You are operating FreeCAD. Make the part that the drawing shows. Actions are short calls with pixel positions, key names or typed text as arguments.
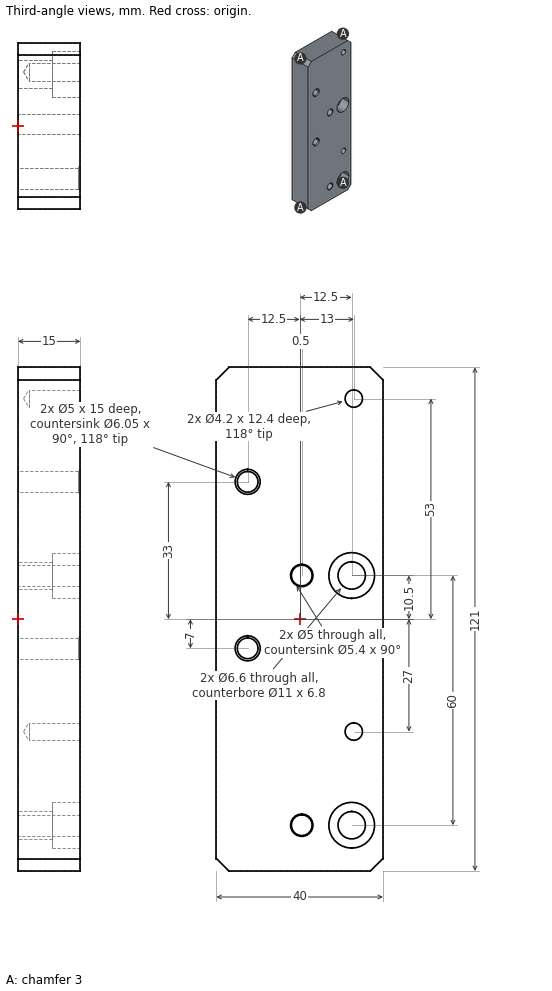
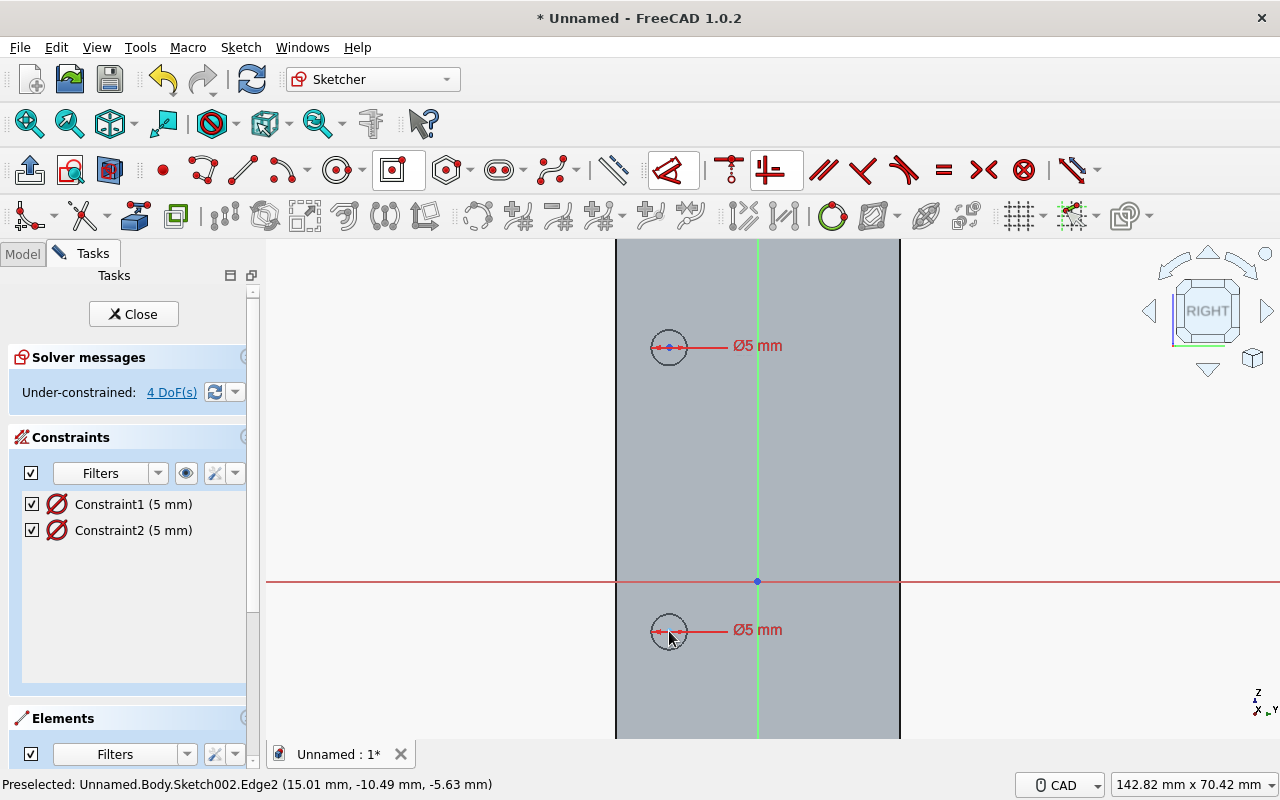
click(669, 348)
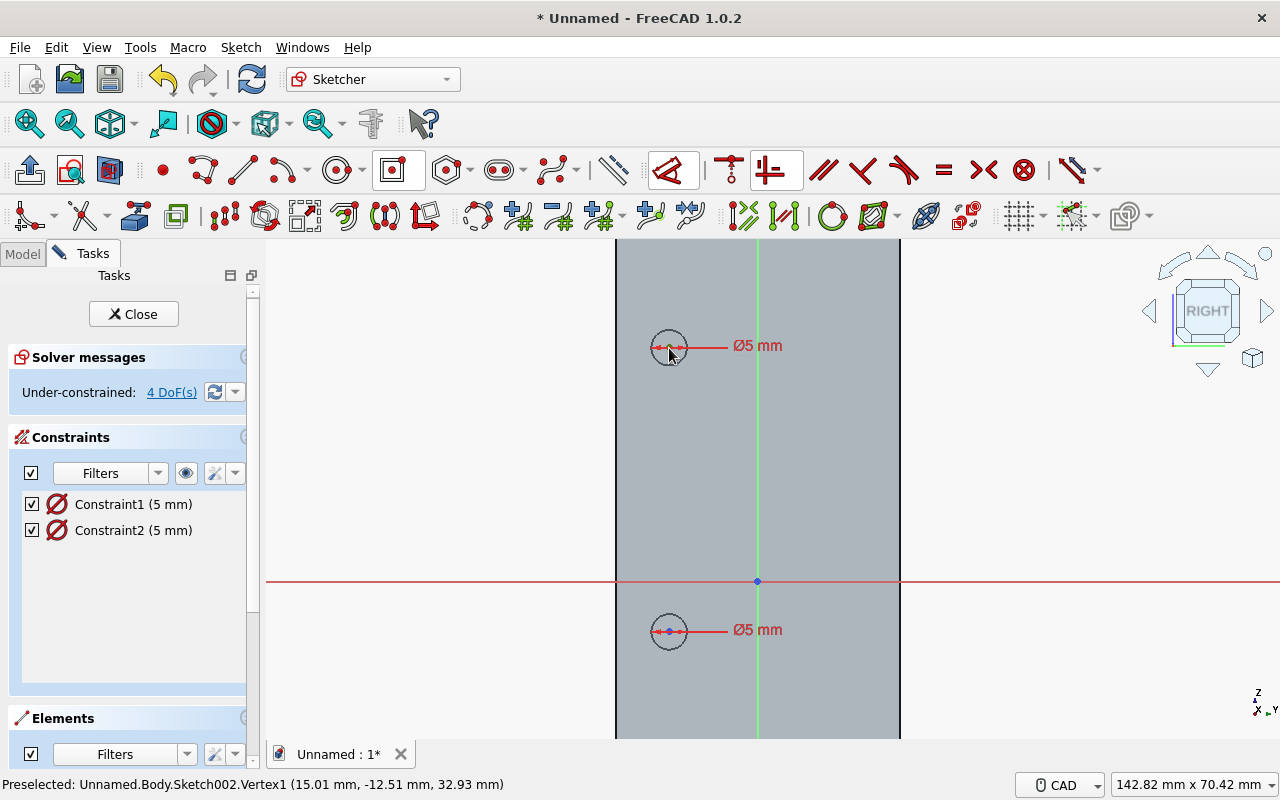
click(669, 632)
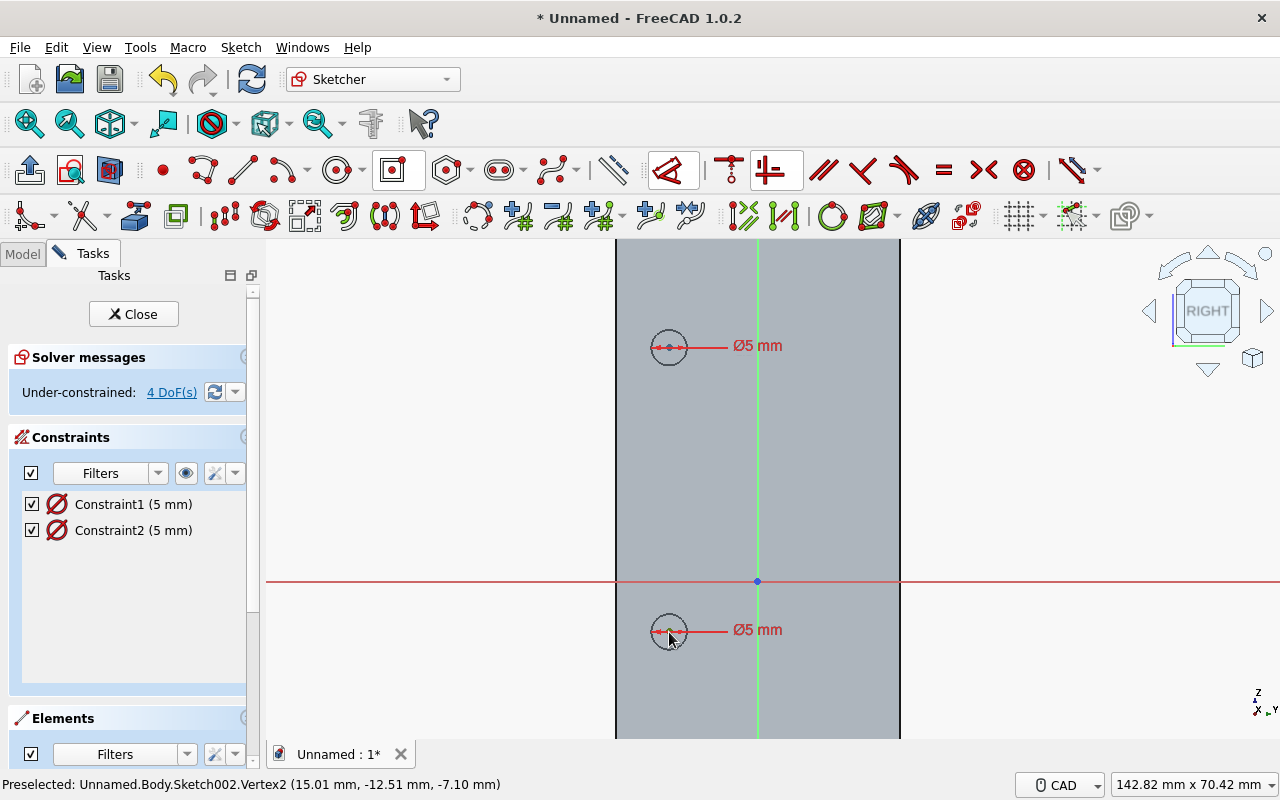
click(798, 170)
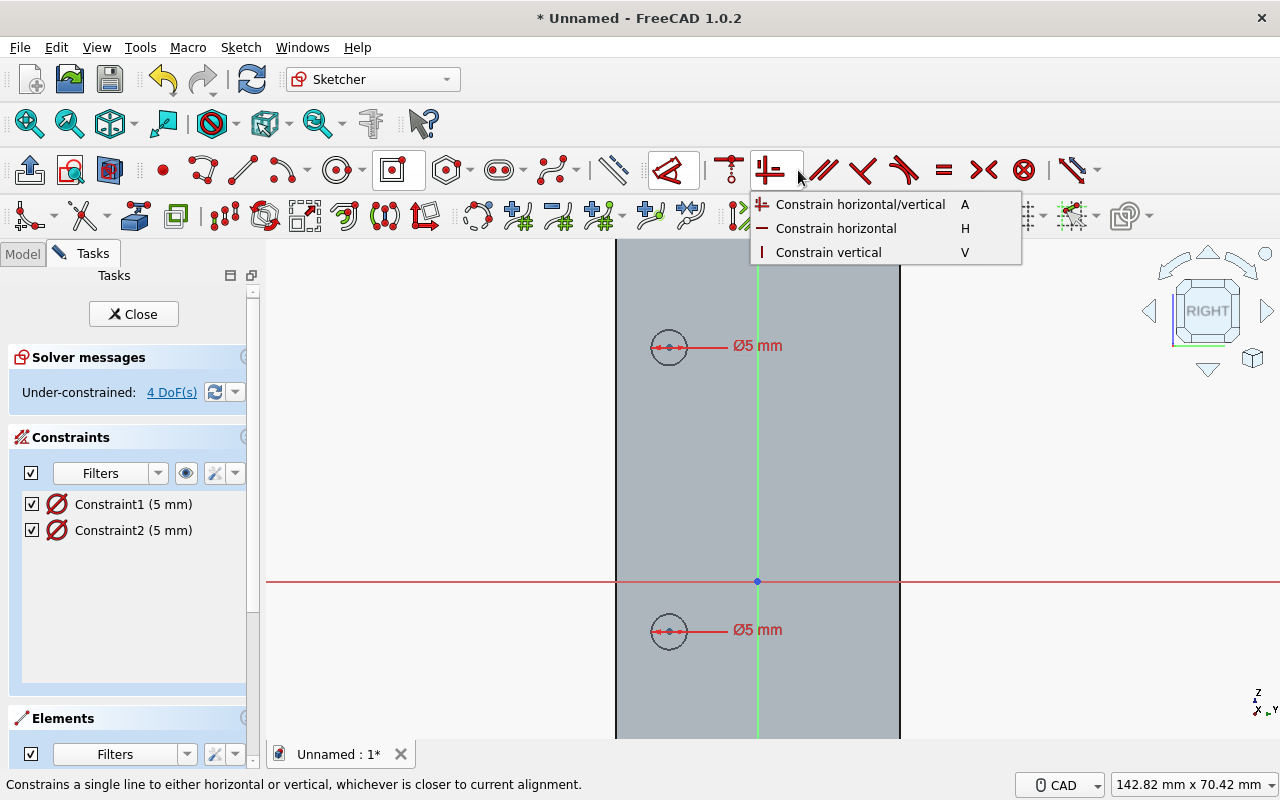
click(886, 252)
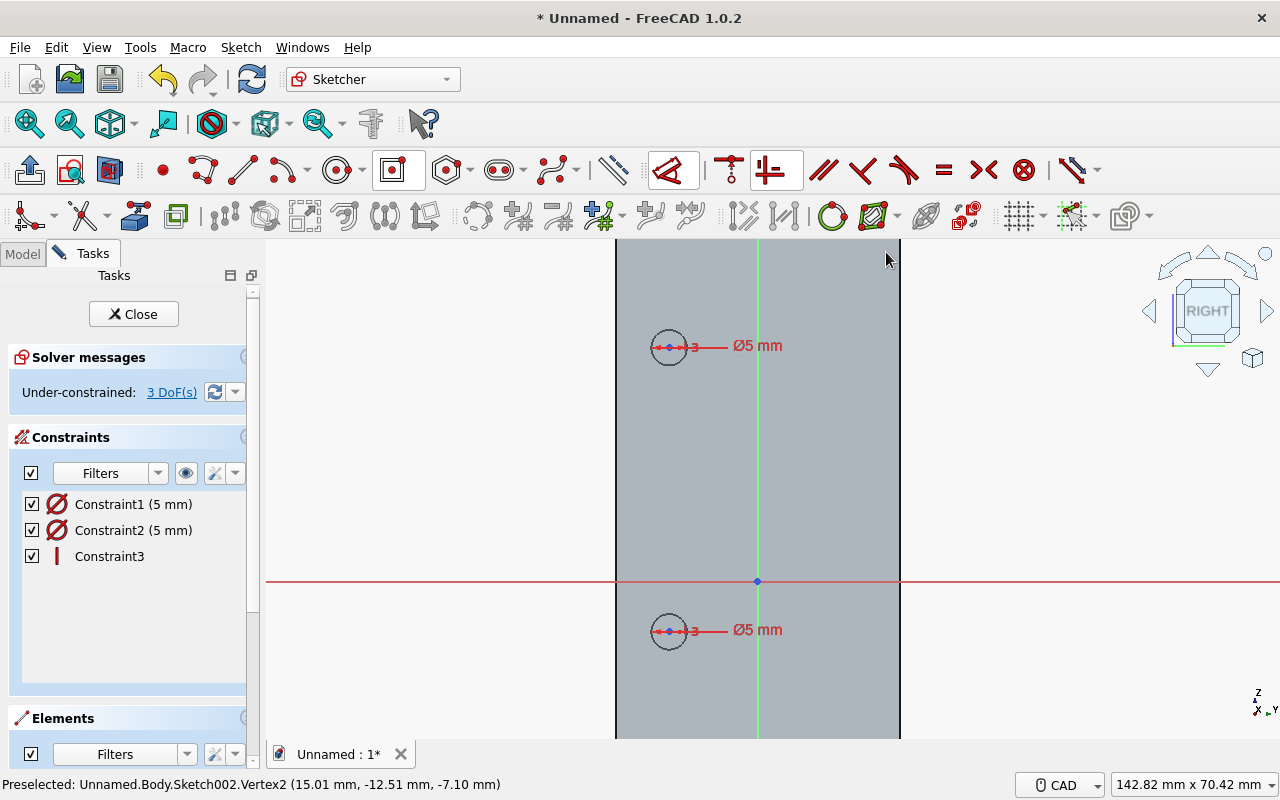
click(669, 632)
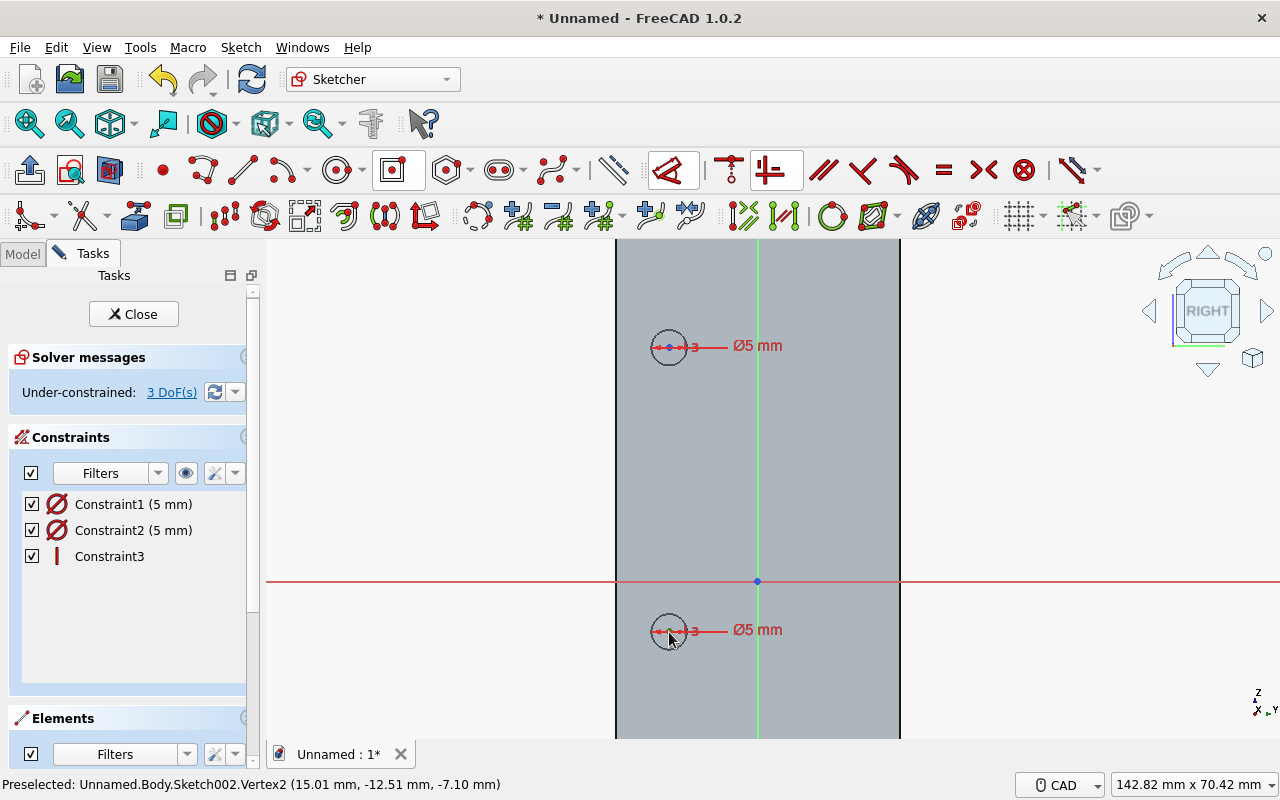
key(i)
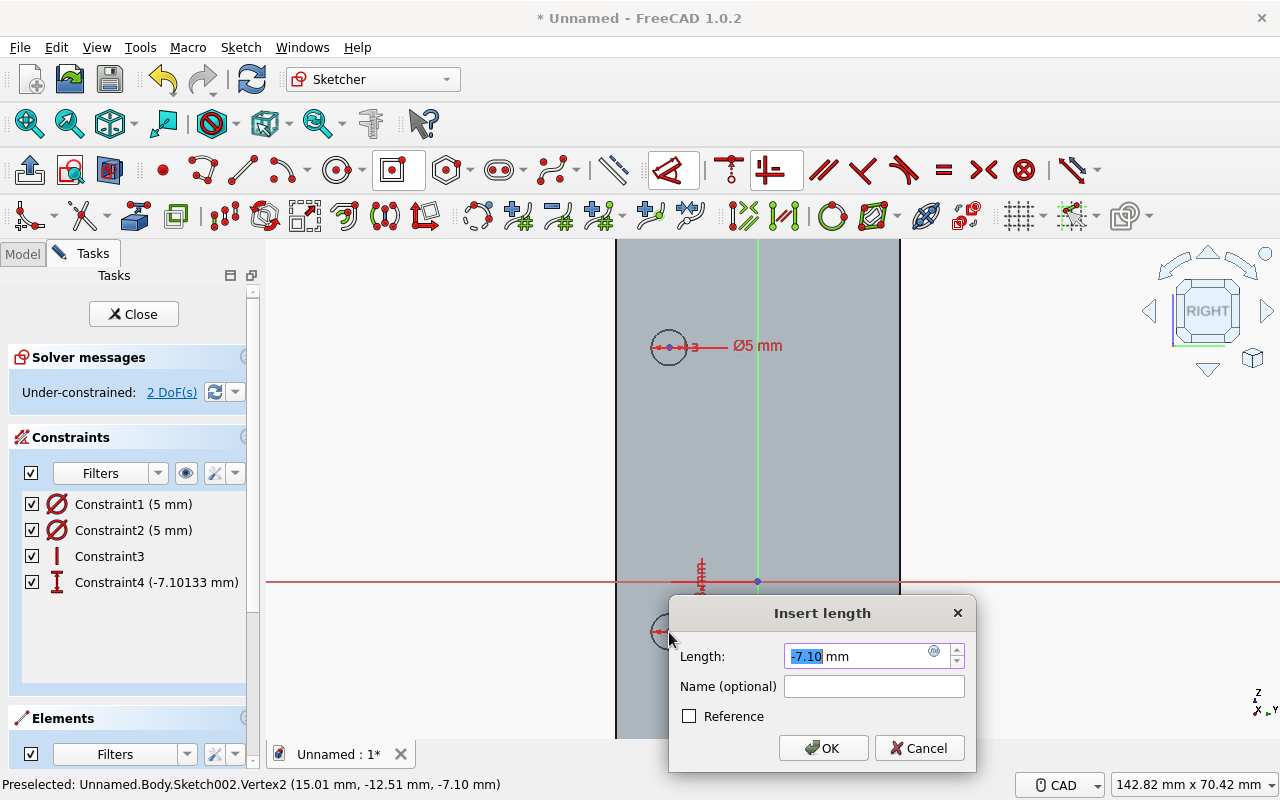
text(-7)
key(Return)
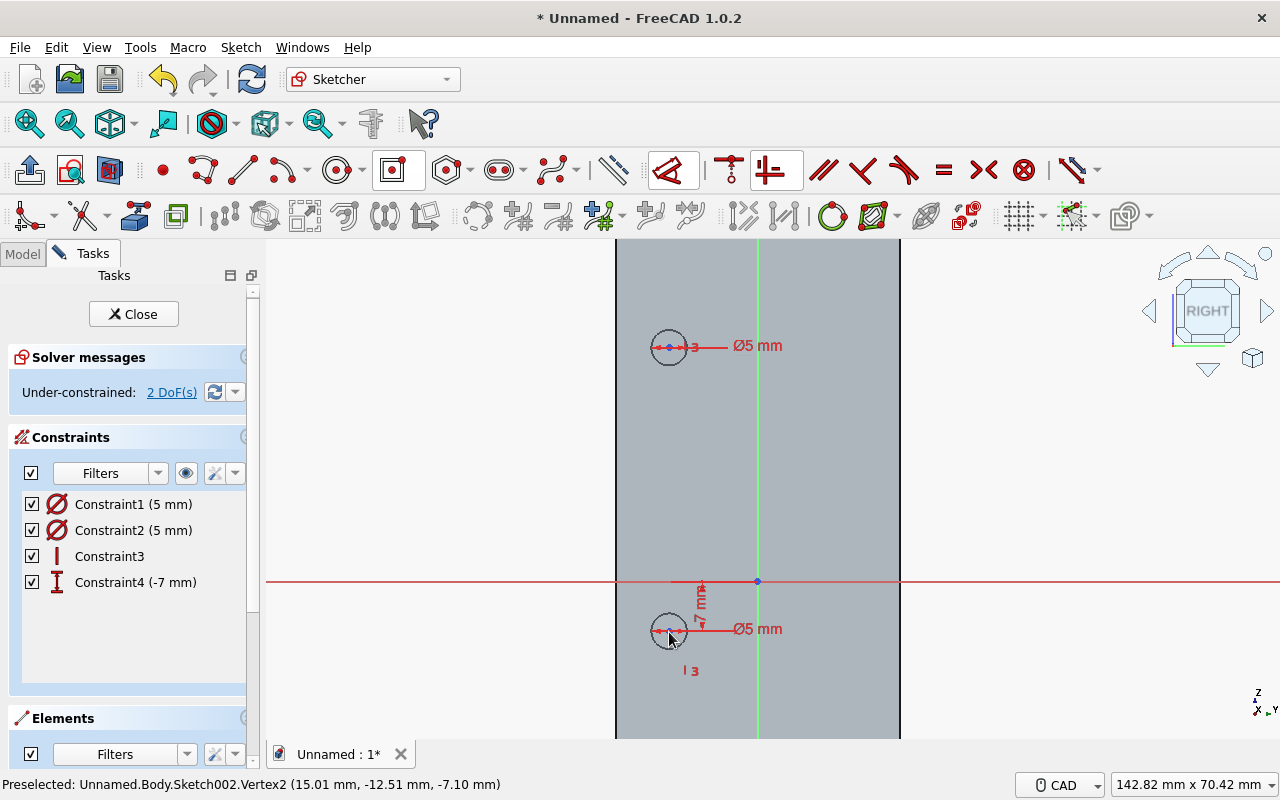
click(669, 348)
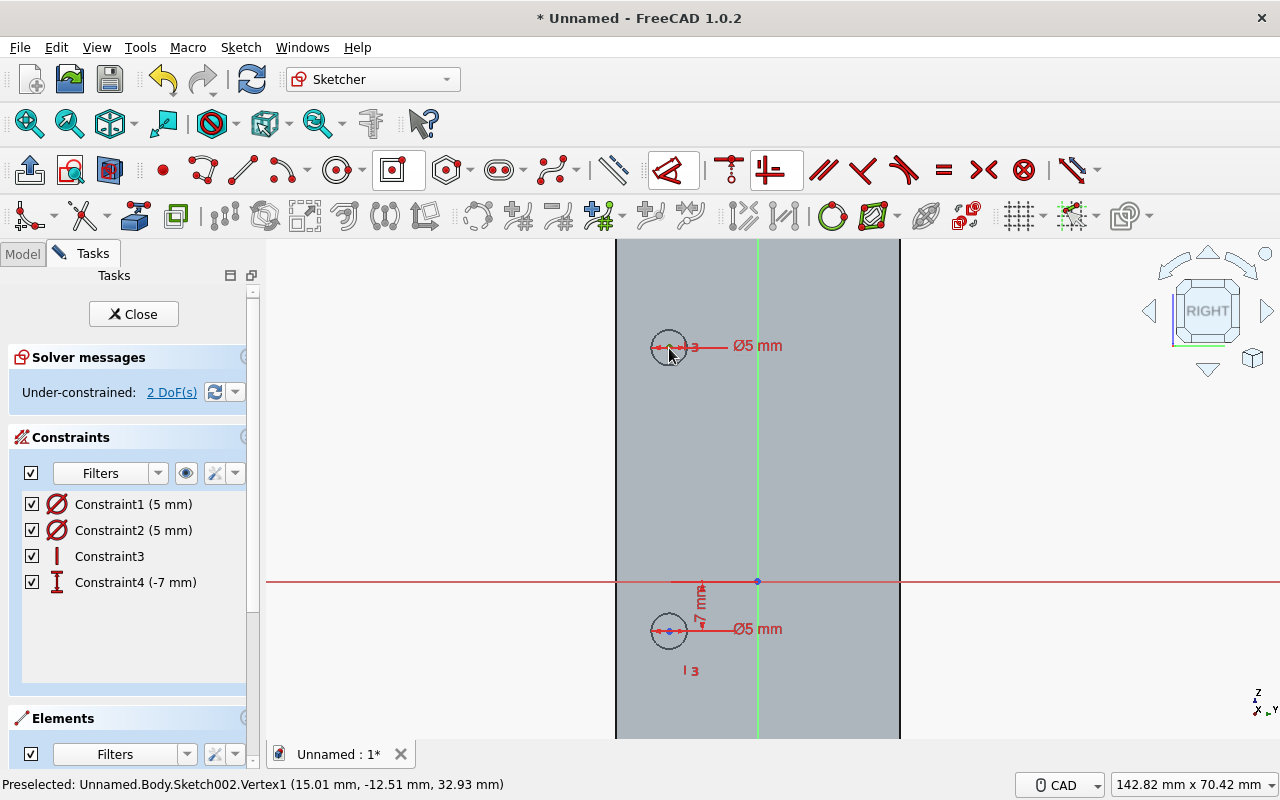
click(694, 170)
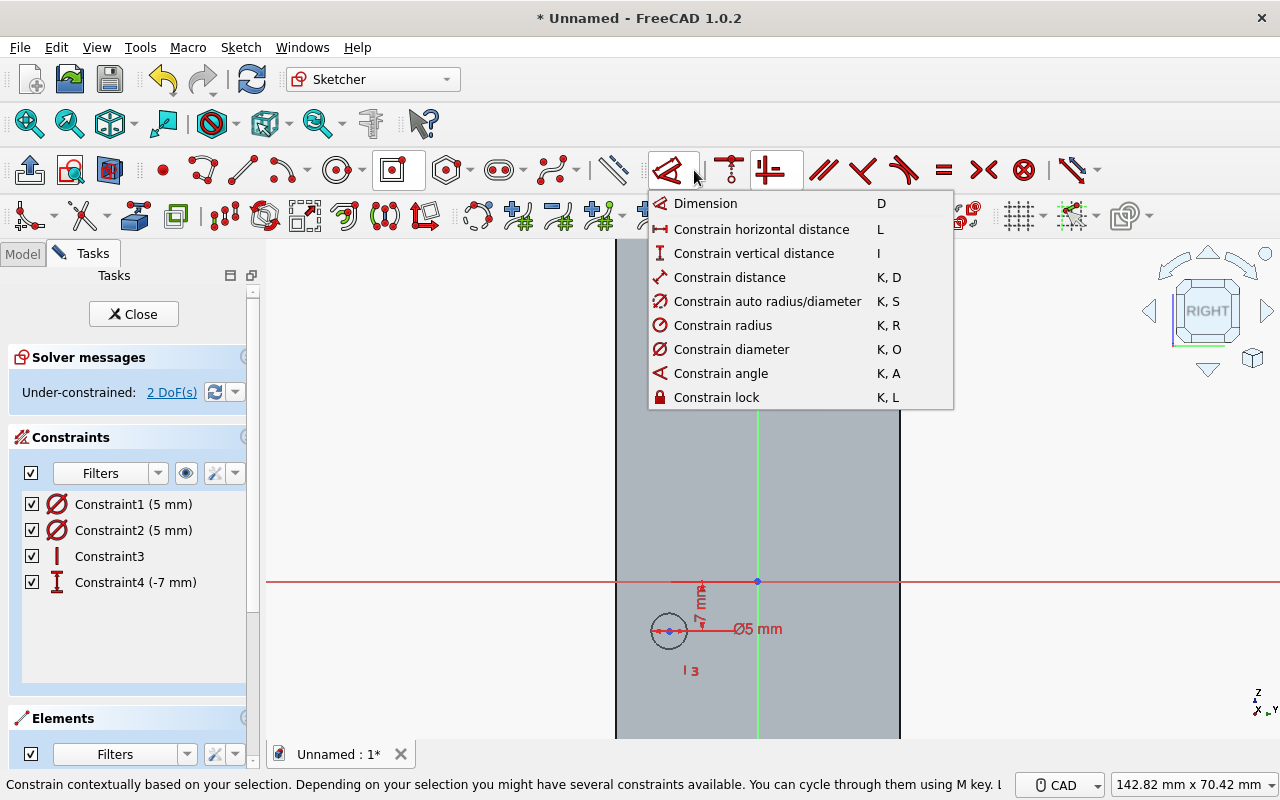
click(801, 253)